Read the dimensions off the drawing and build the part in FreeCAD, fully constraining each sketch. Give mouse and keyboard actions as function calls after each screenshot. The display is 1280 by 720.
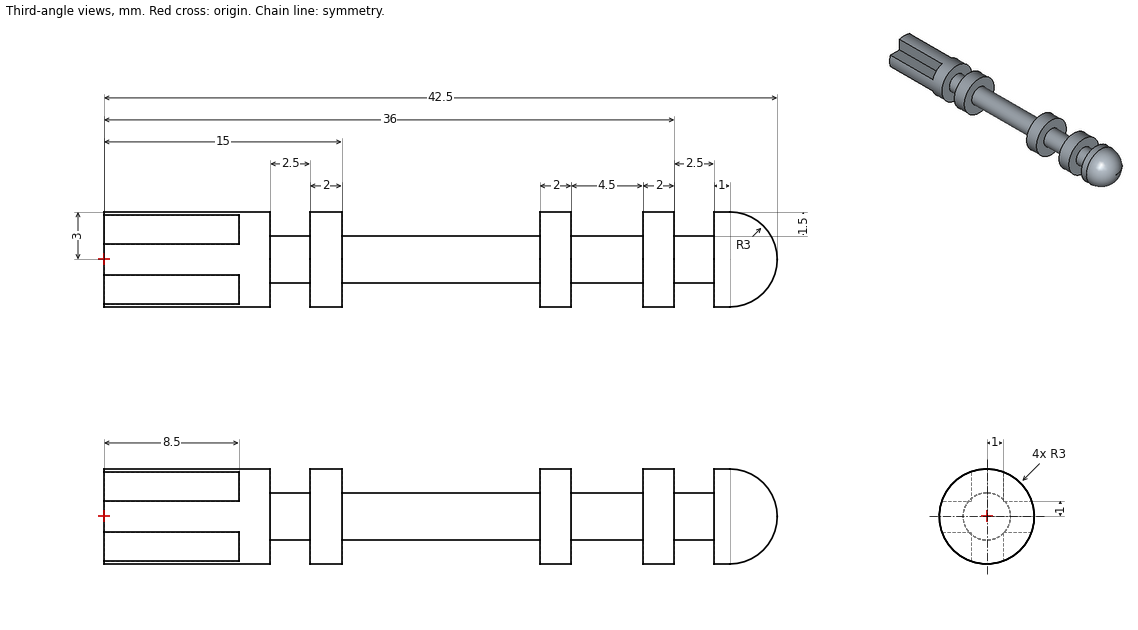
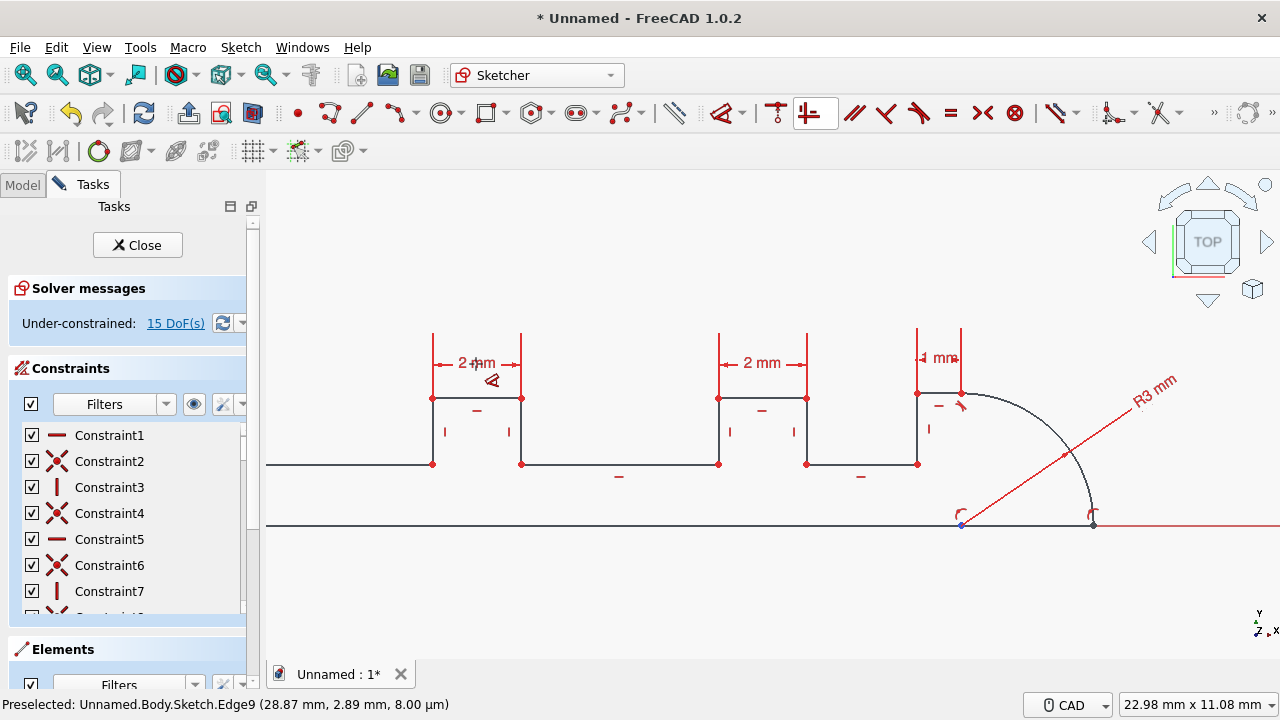
scroll(941, 395, down, 6)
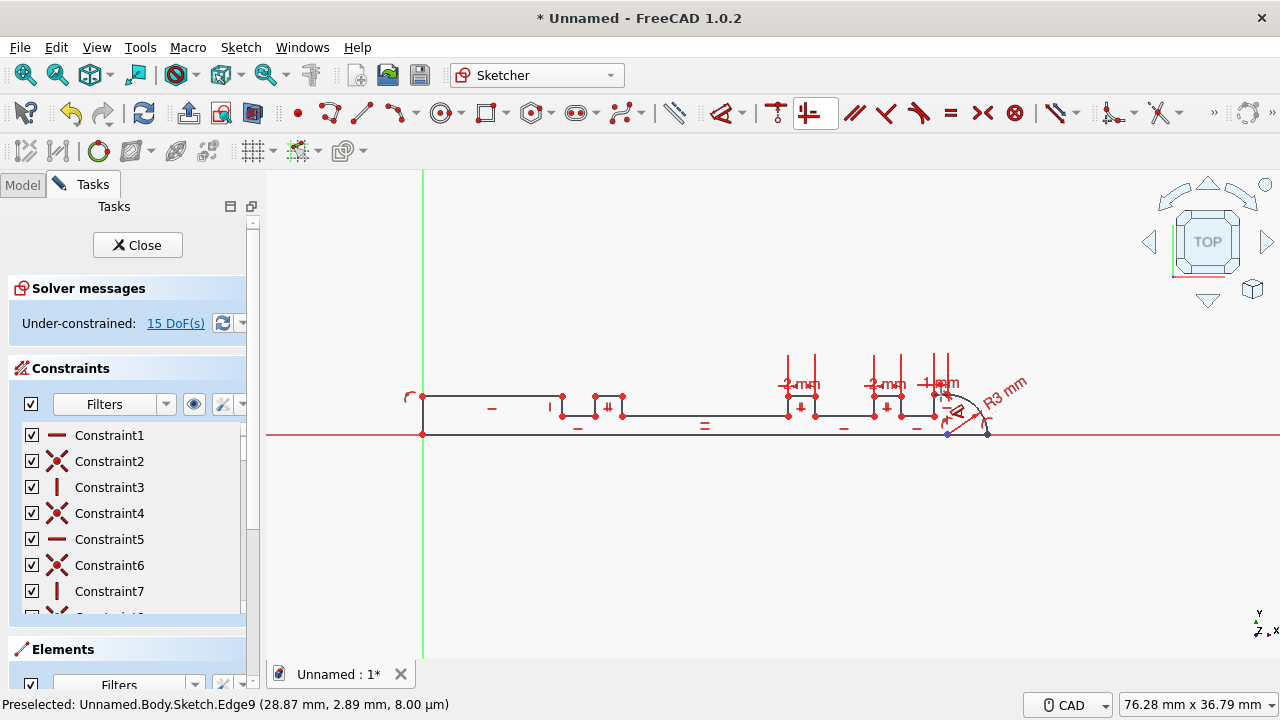
scroll(614, 396, up, 3)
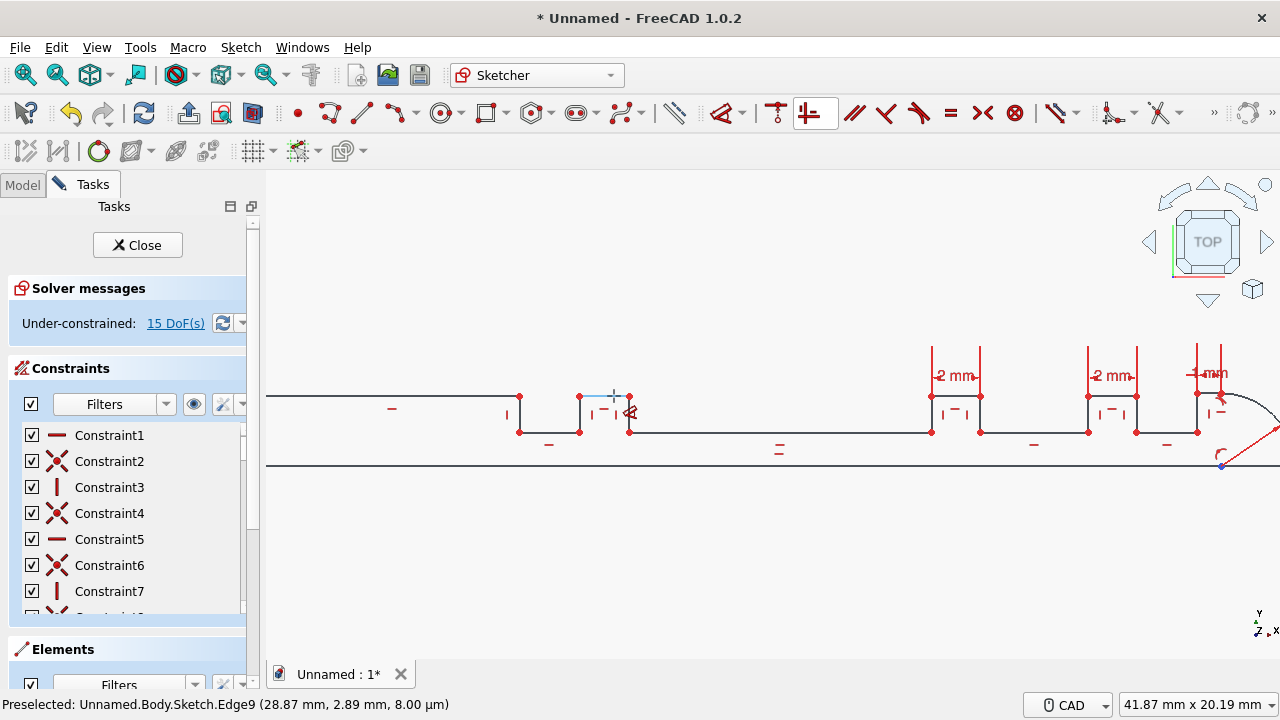
click(614, 396)
click(605, 362)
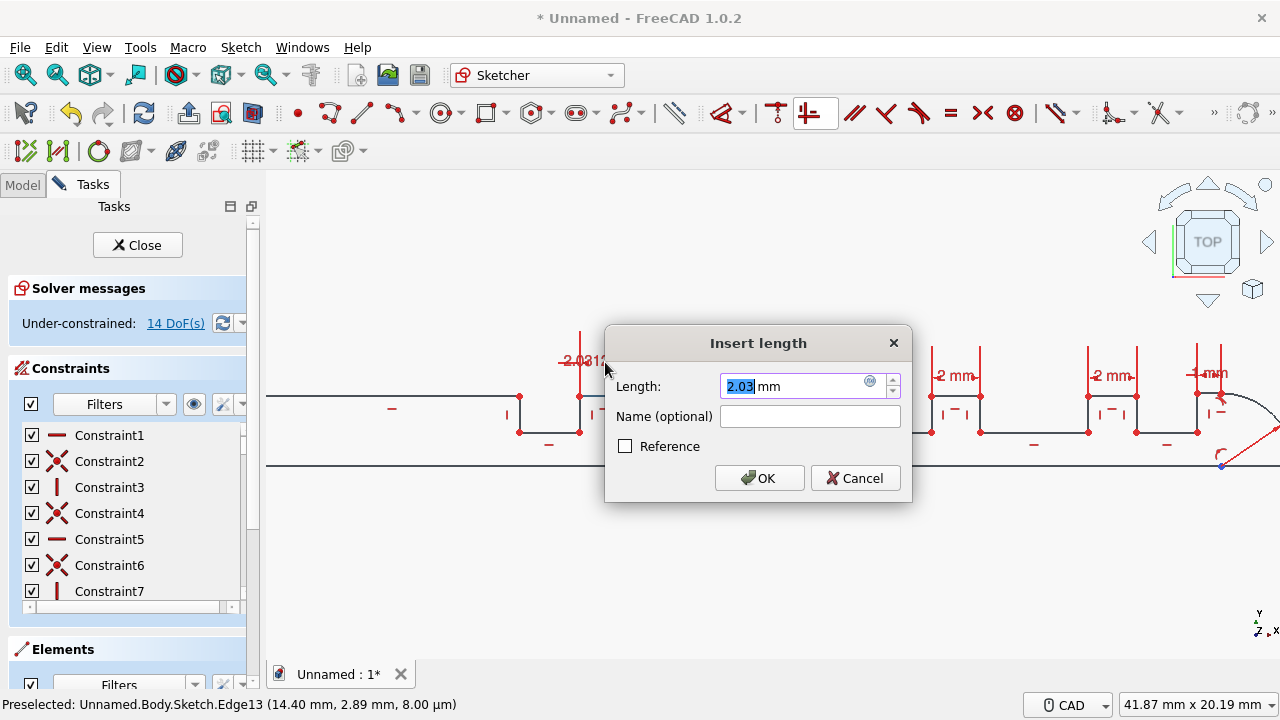
text(2)
key(Return)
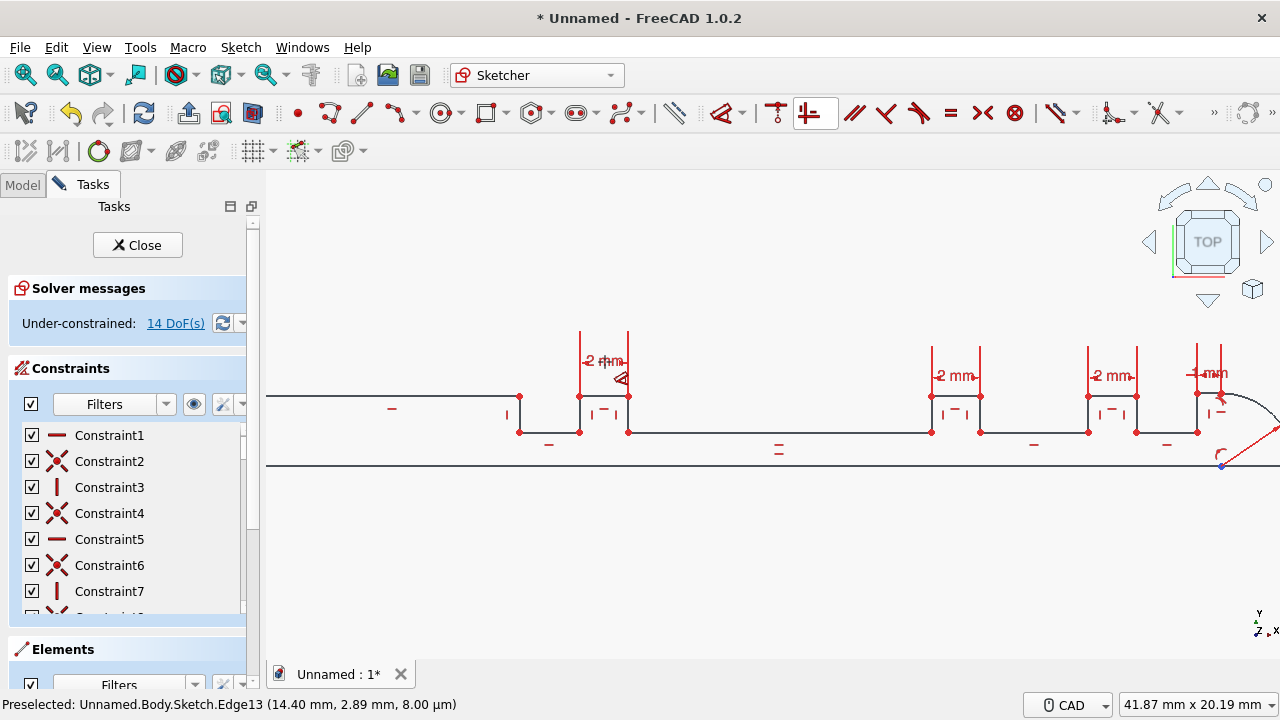
scroll(613, 396, down, 3)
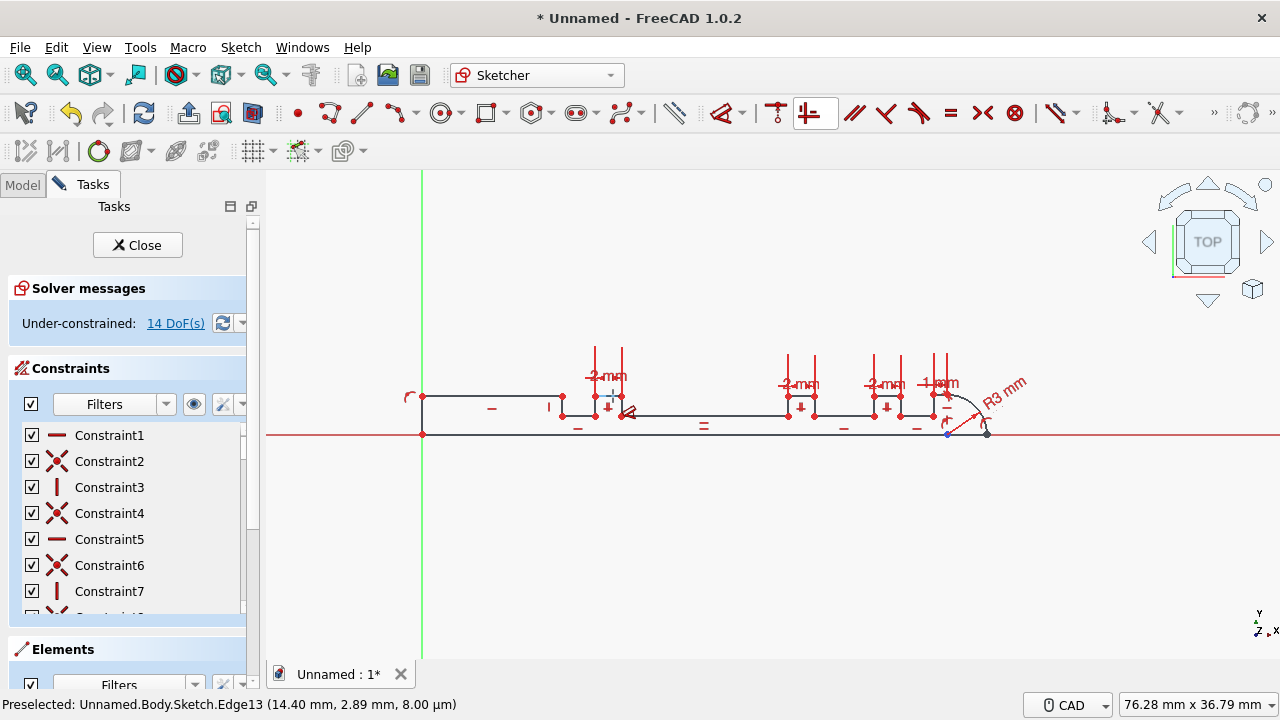
click(422, 408)
click(388, 415)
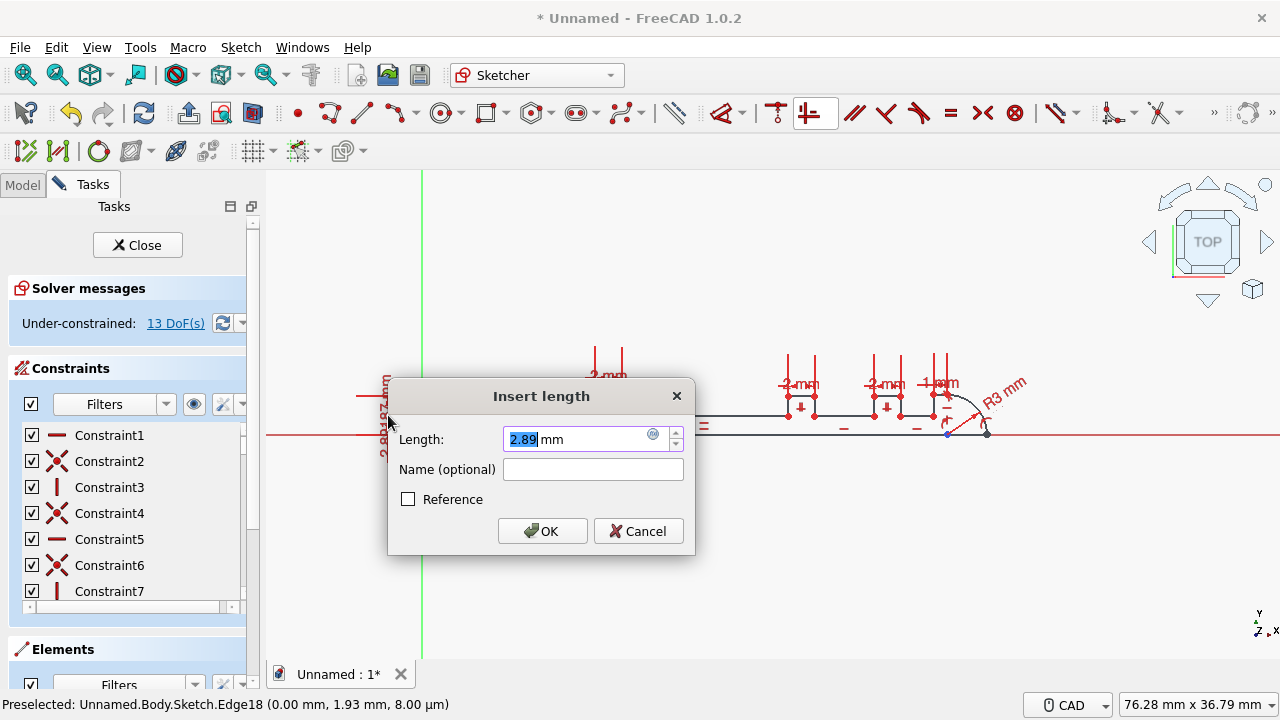
text(3)
key(Return)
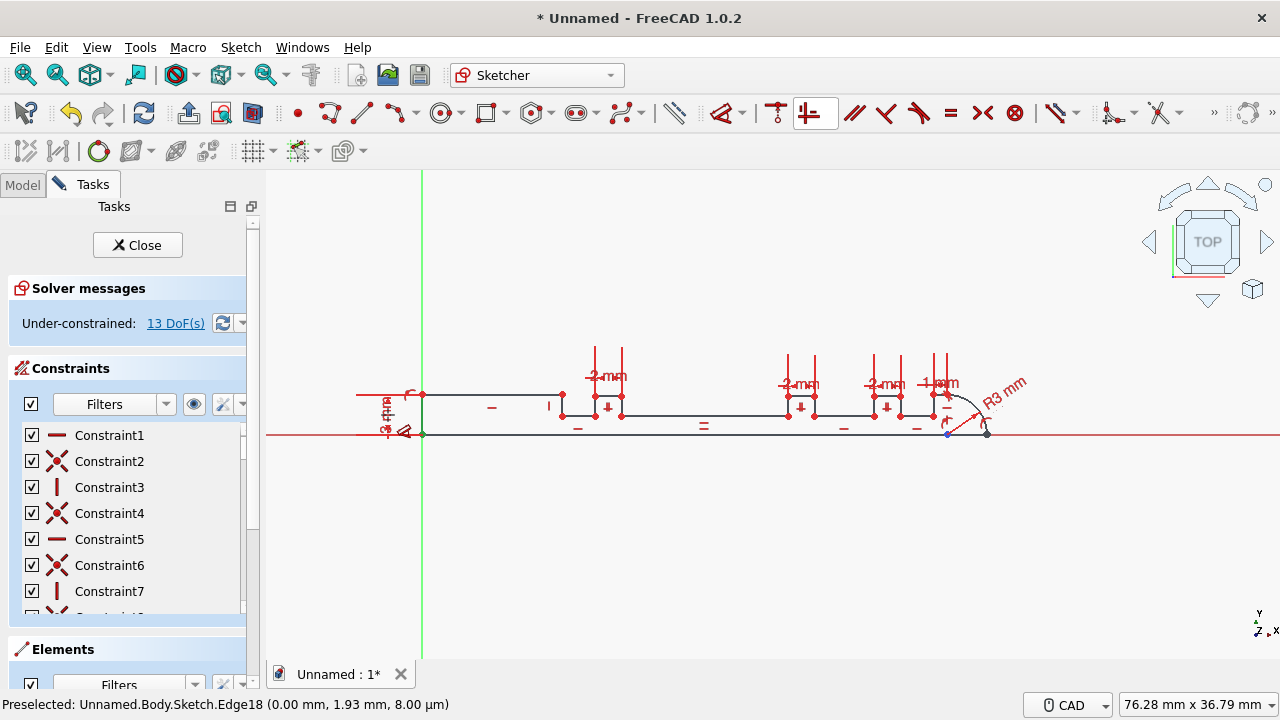
click(901, 396)
click(959, 415)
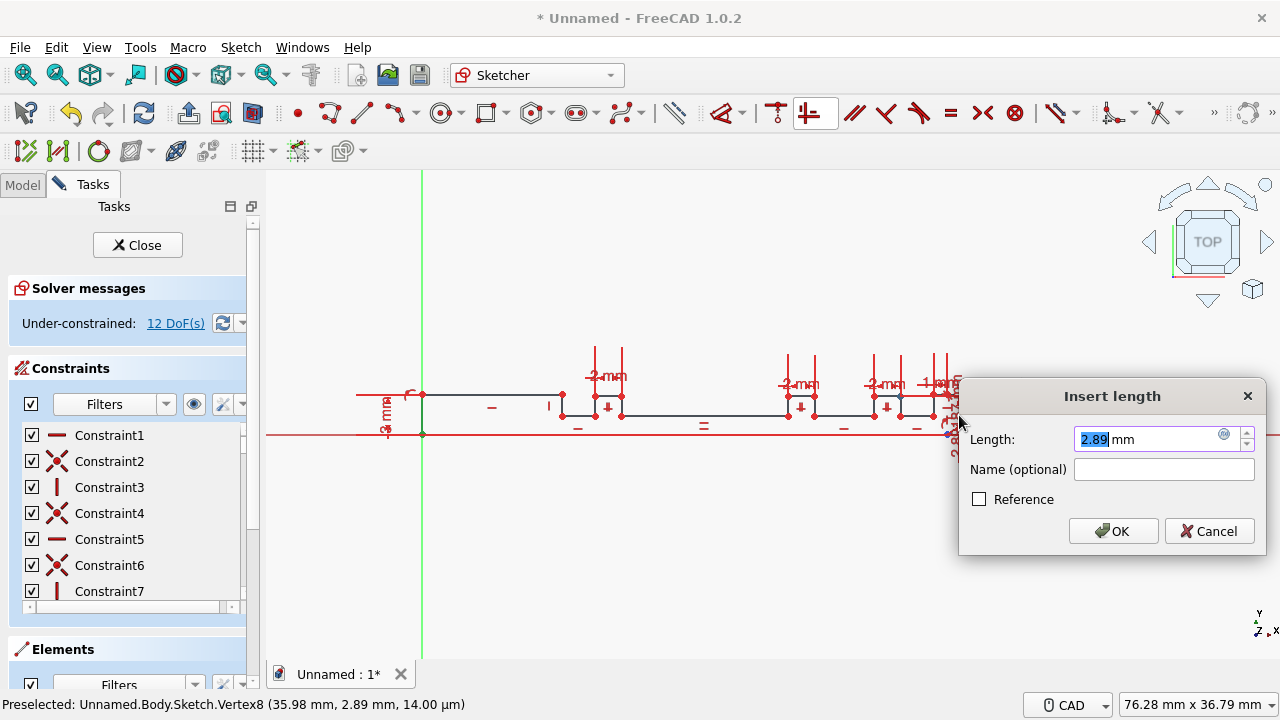
text(3)
key(Return)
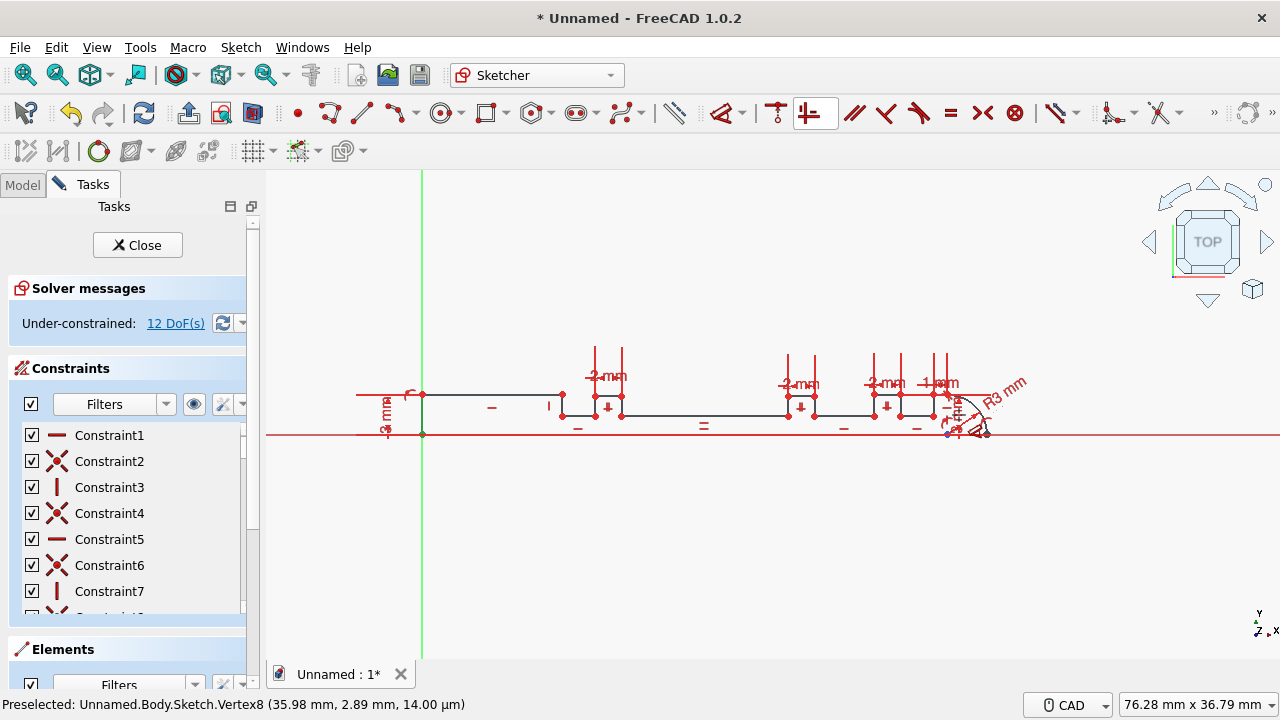
click(815, 396)
click(316, 415)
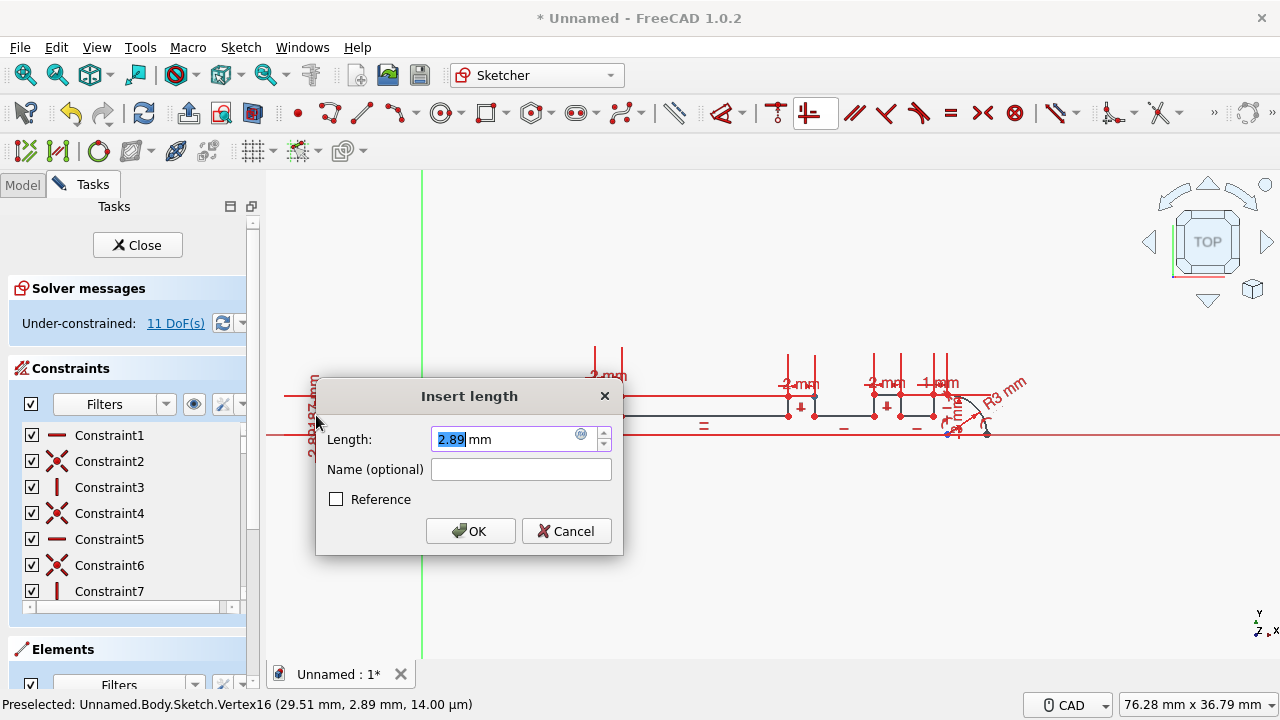
text(3)
key(Return)